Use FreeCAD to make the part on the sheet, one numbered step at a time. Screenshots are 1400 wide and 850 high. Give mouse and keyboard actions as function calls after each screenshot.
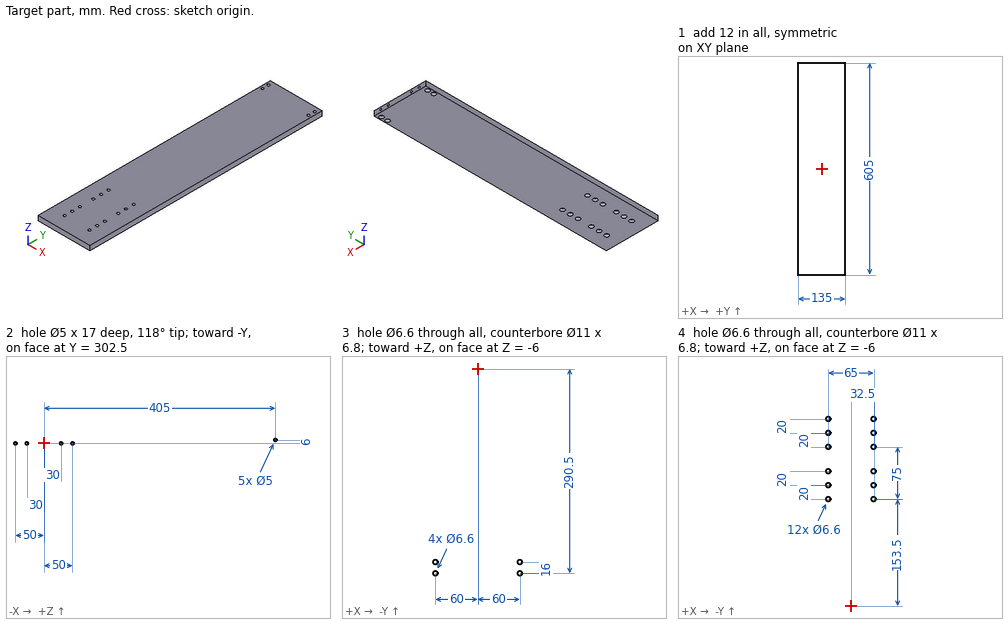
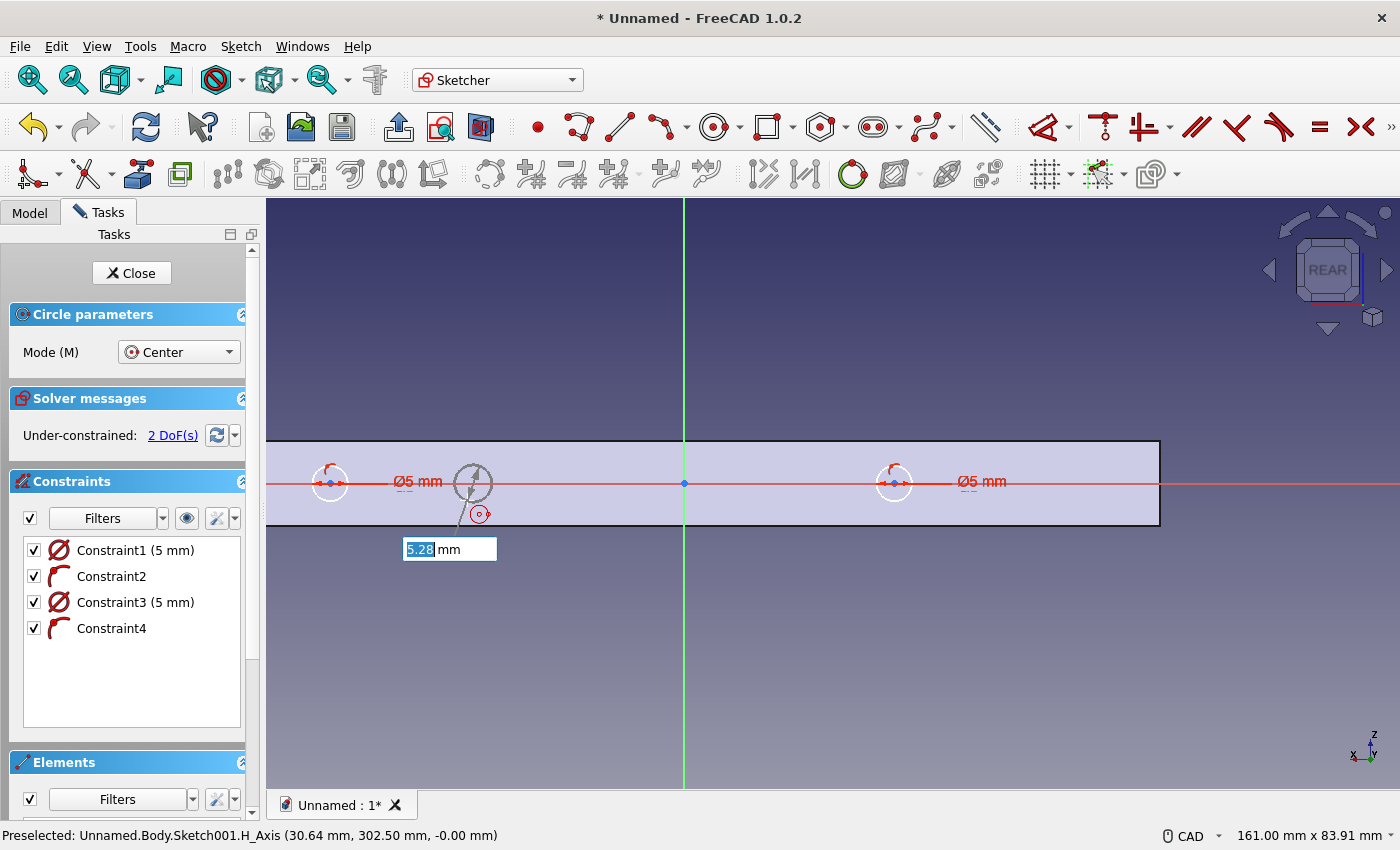
text(5)
key(Return)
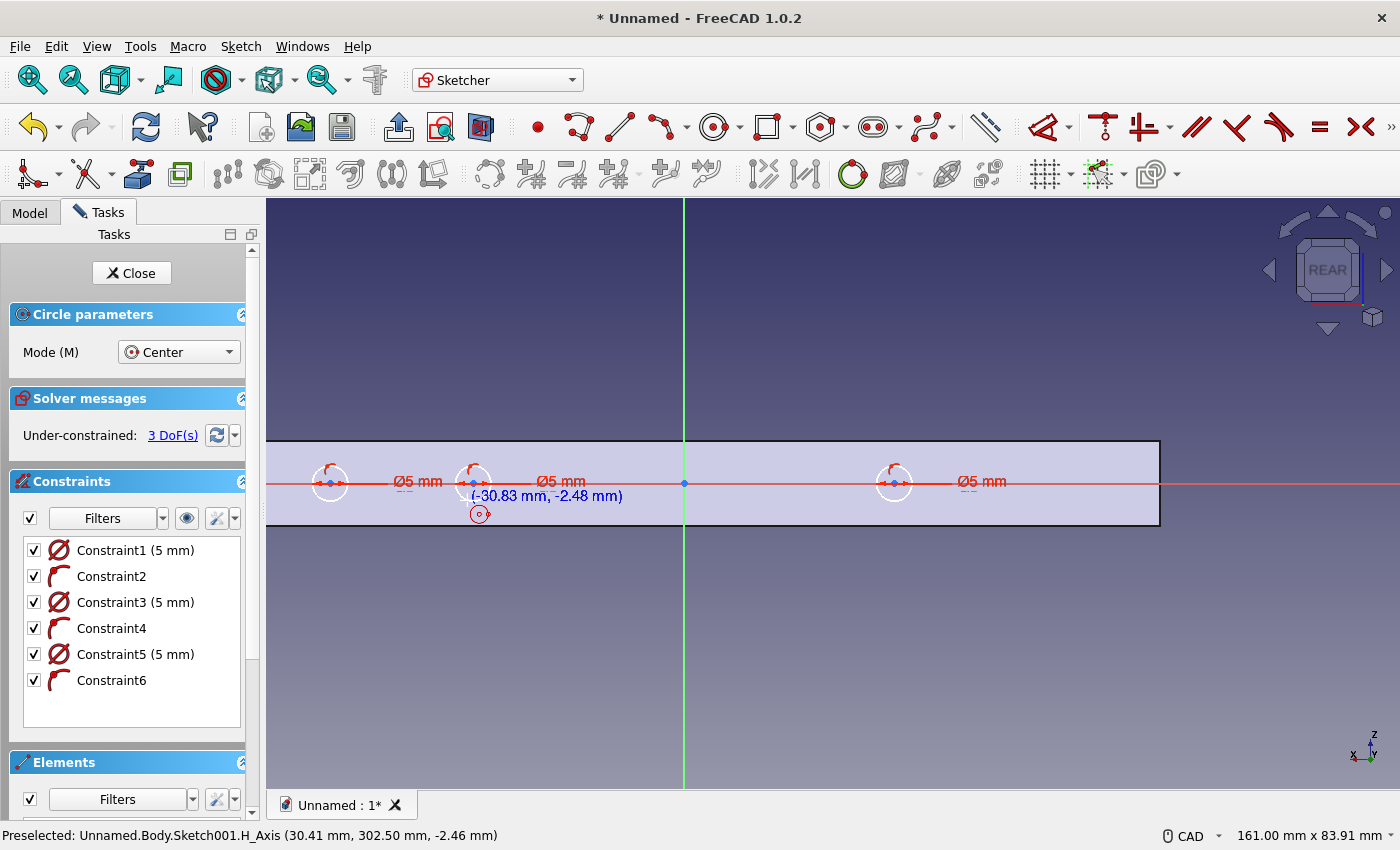
scroll(469, 501, down, 8)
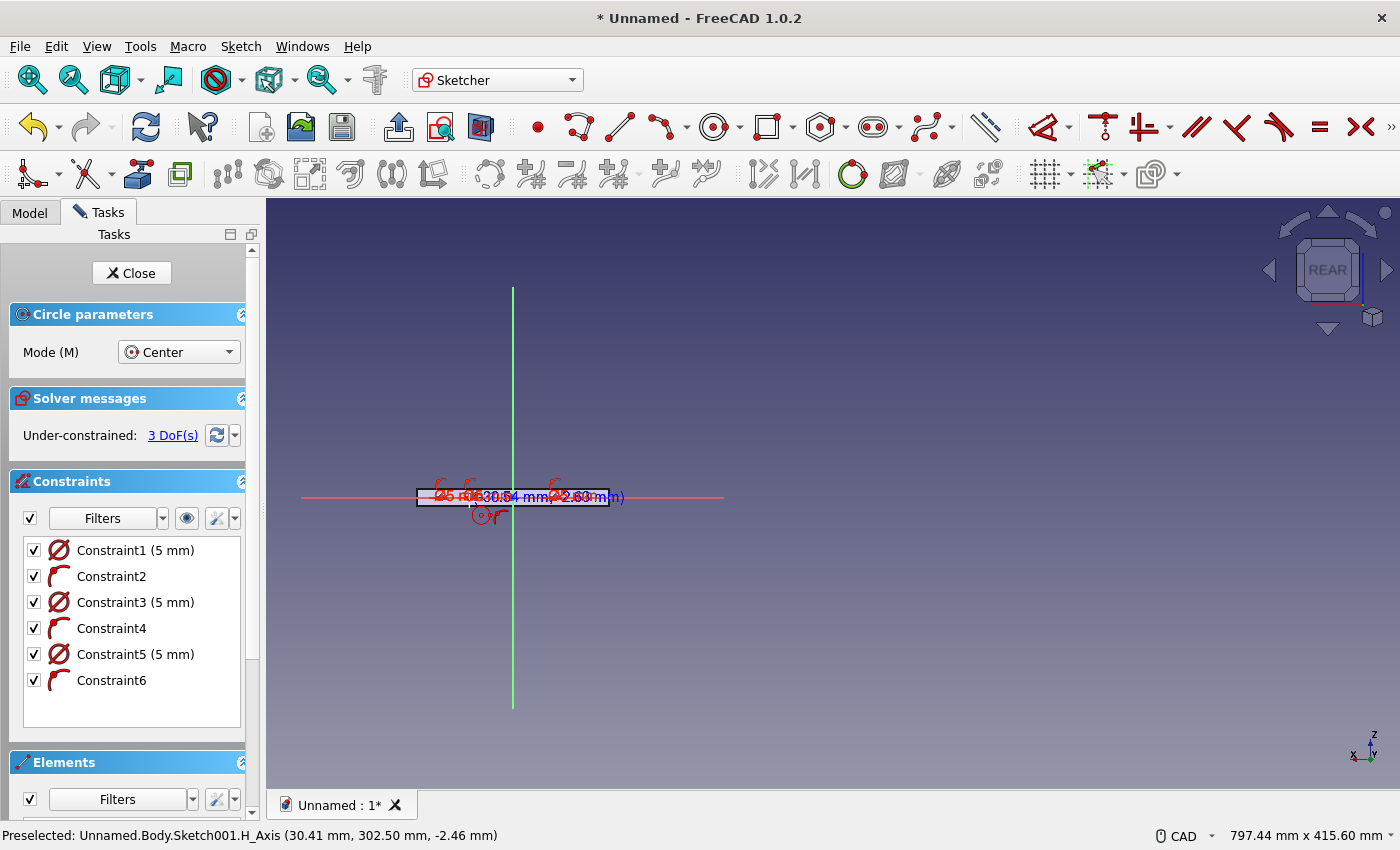
scroll(1089, 489, up, 10)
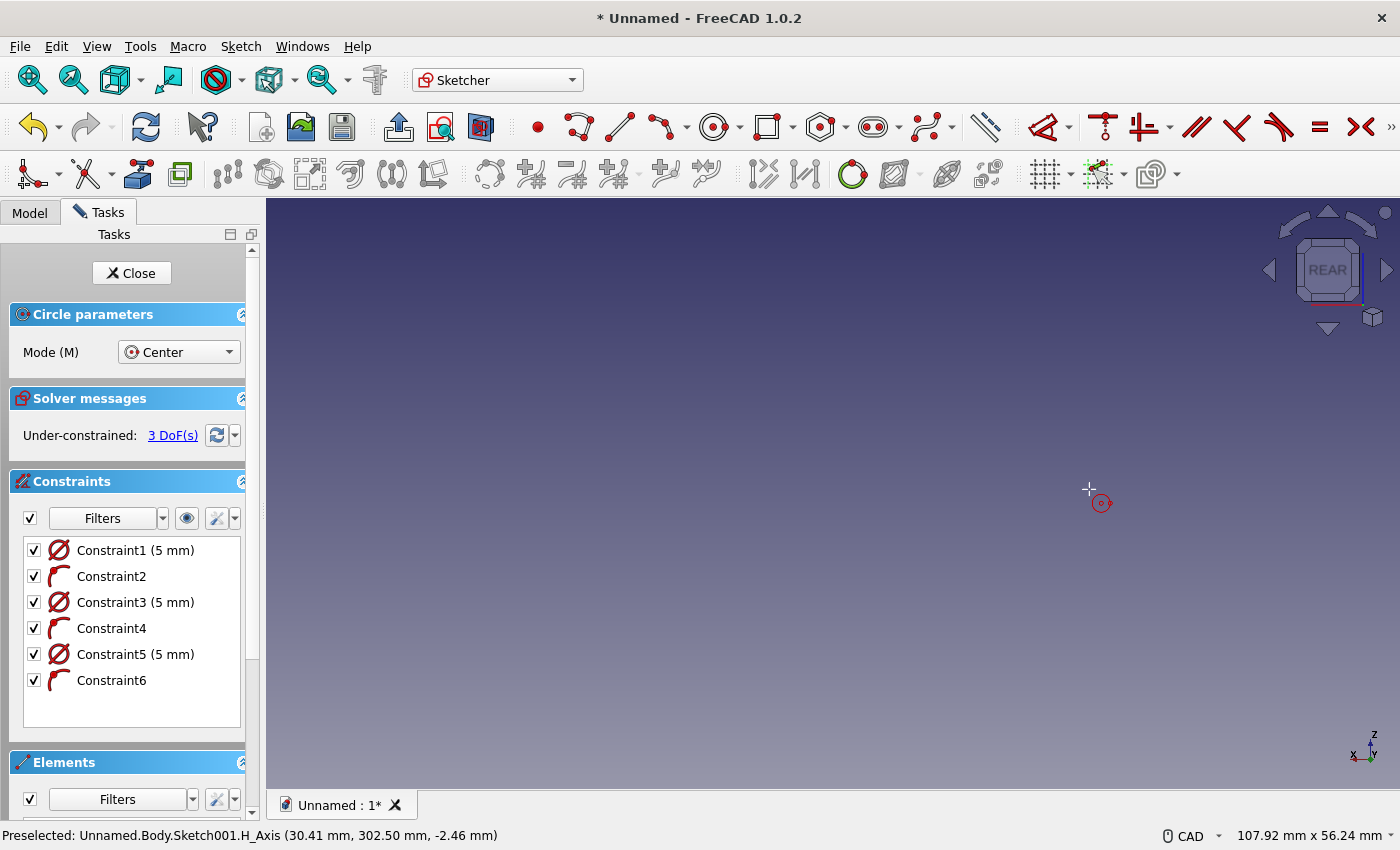
scroll(1089, 489, down, 10)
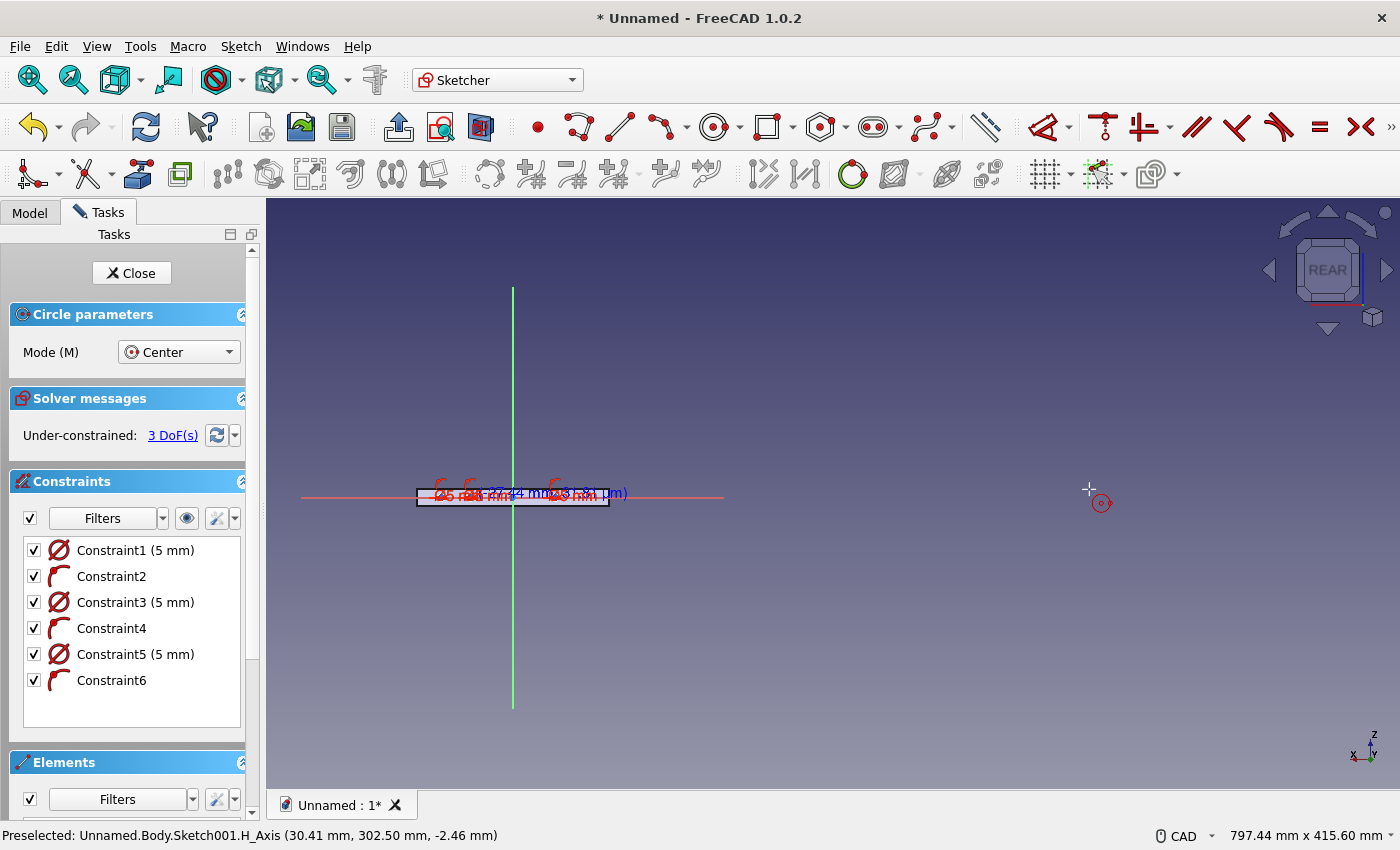
scroll(1089, 489, up, 4)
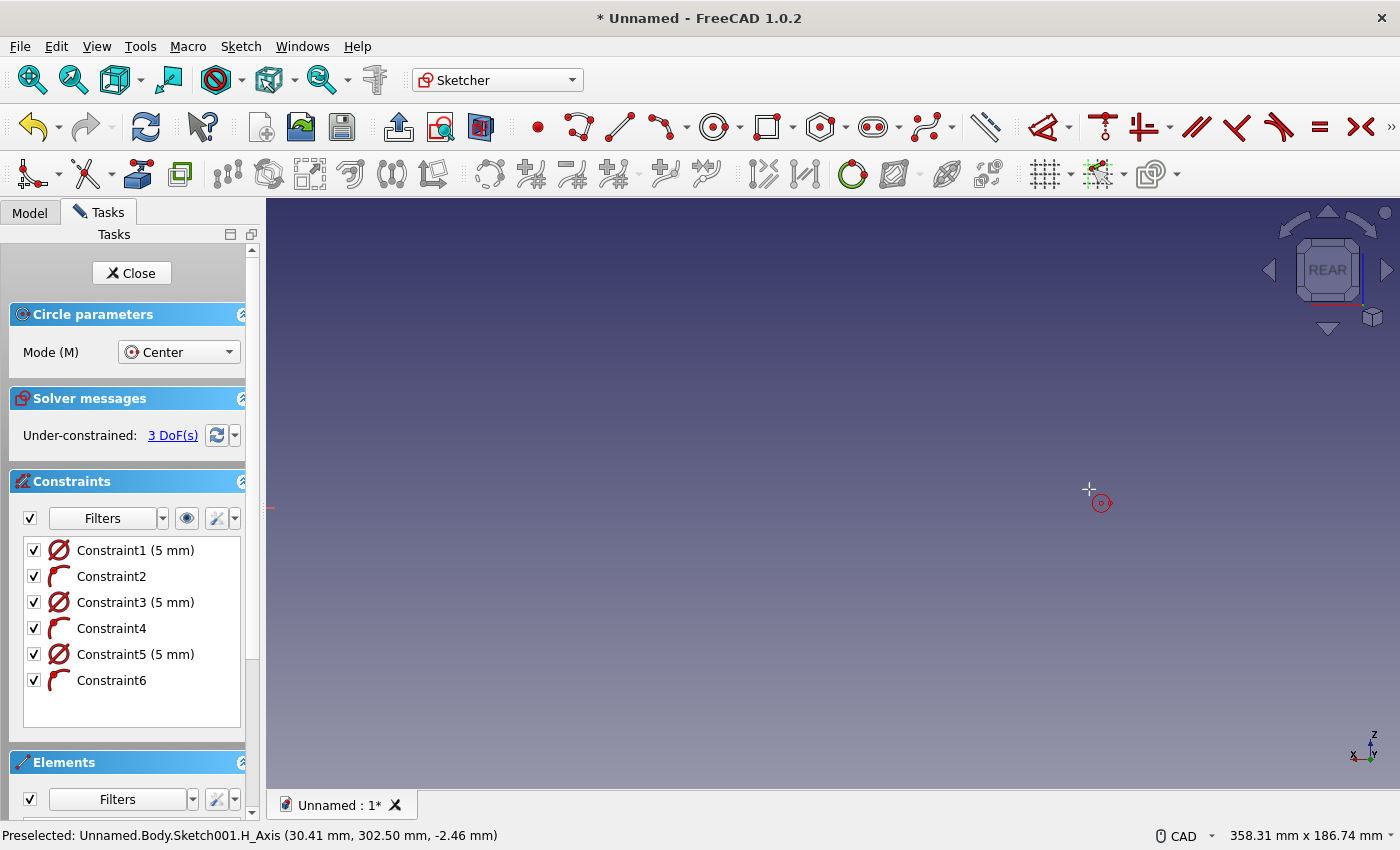
click(1087, 489)
move(1093, 484)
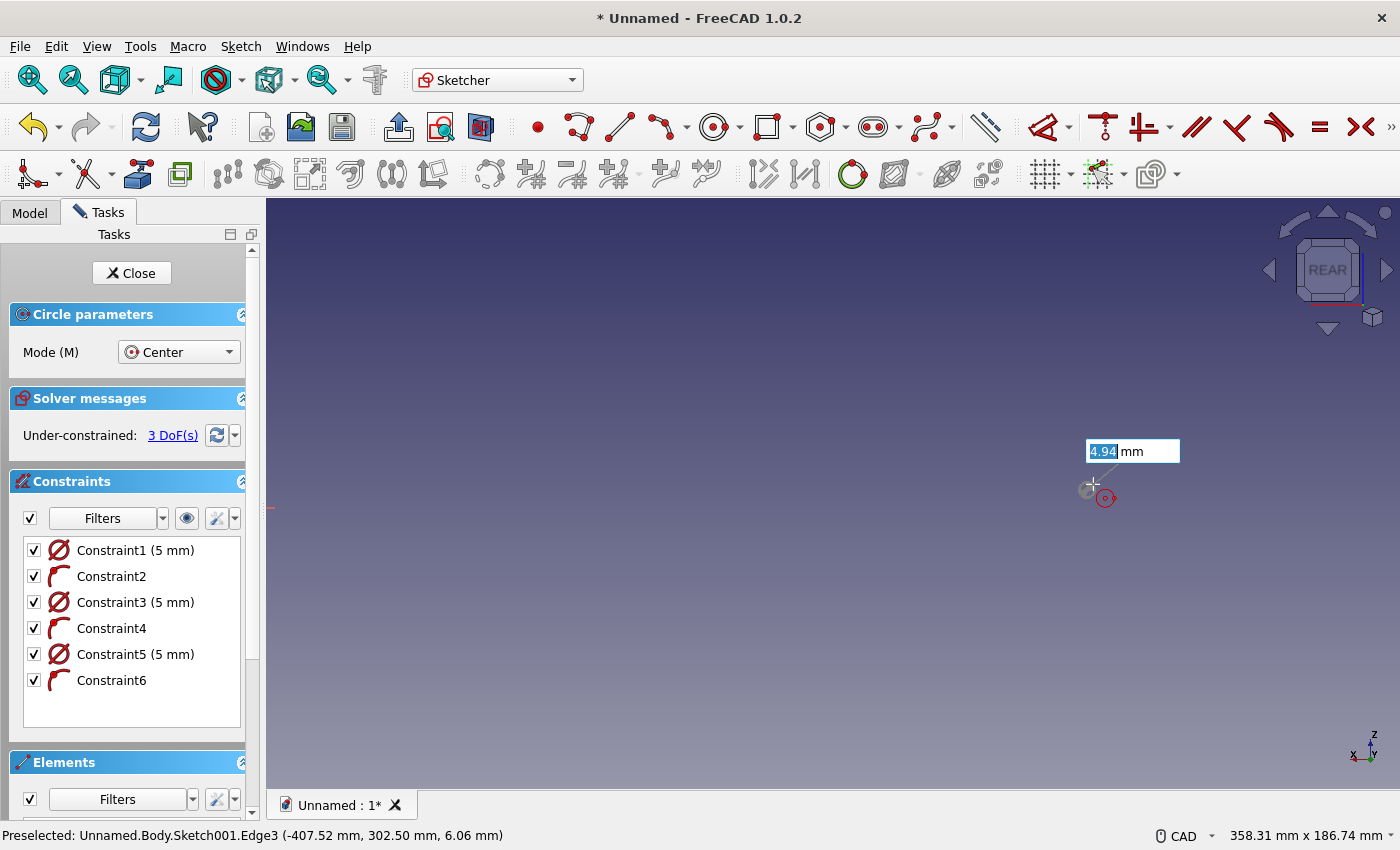
text(5)
key(Return)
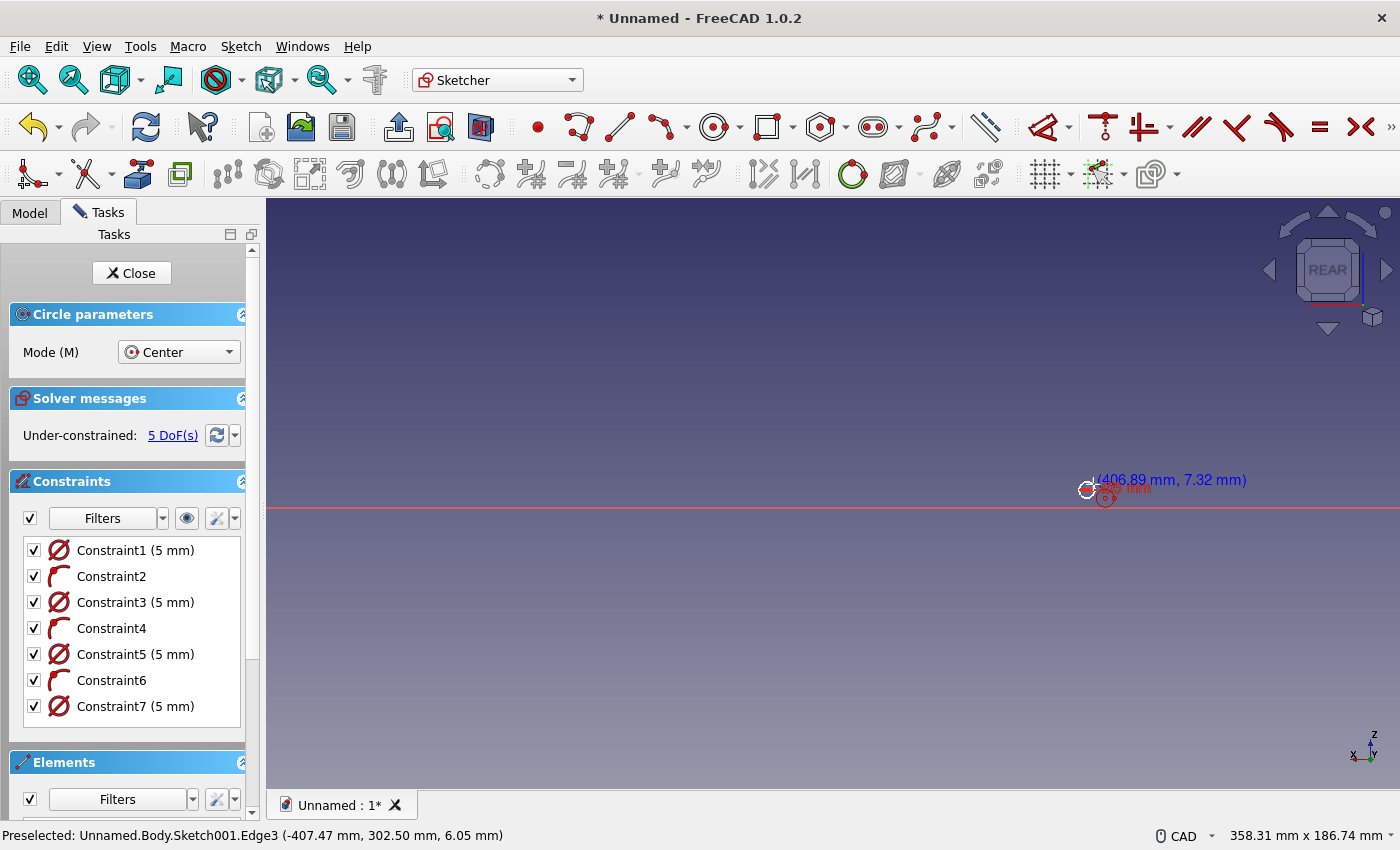
scroll(1089, 489, down, 4)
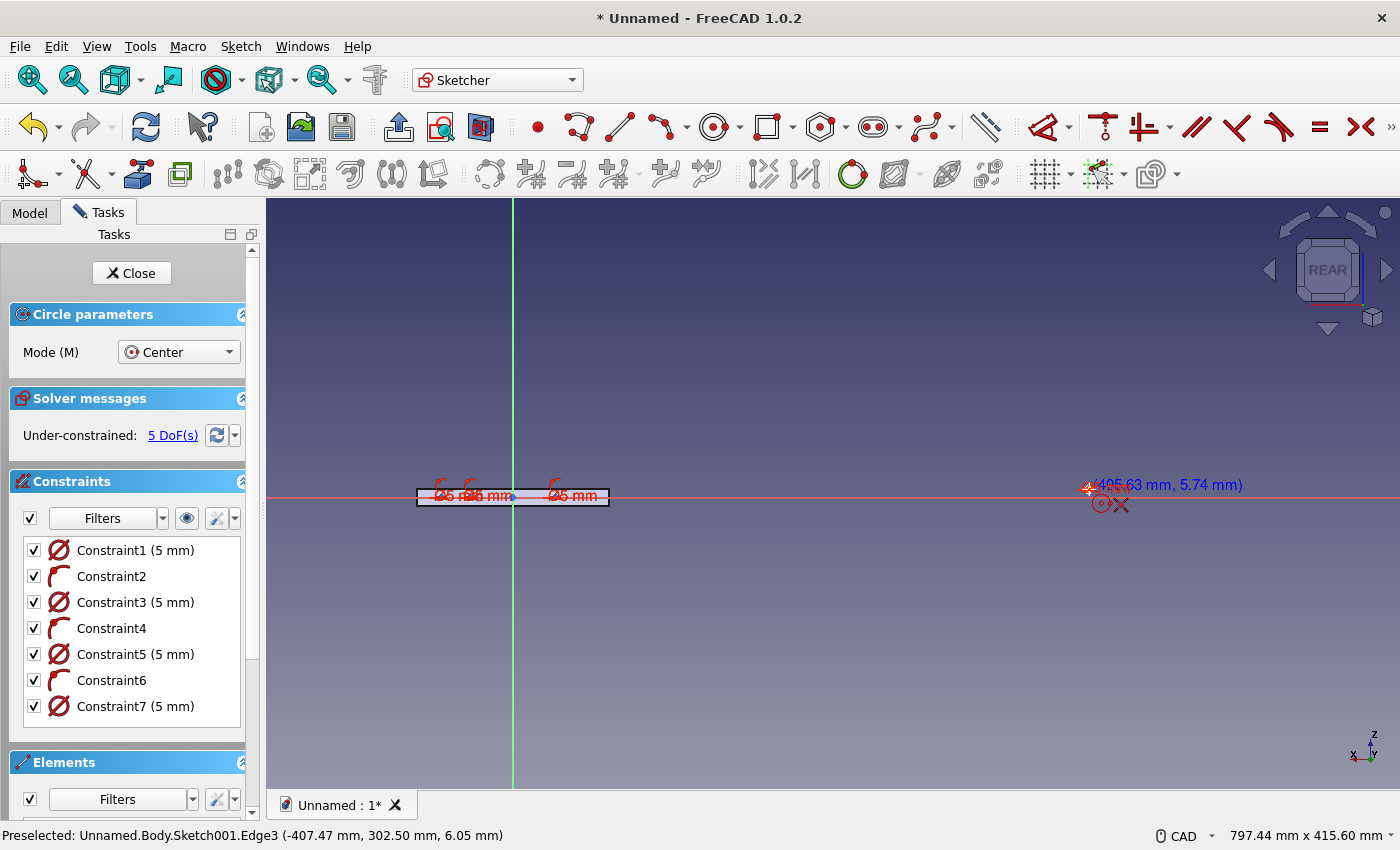
scroll(584, 498, up, 10)